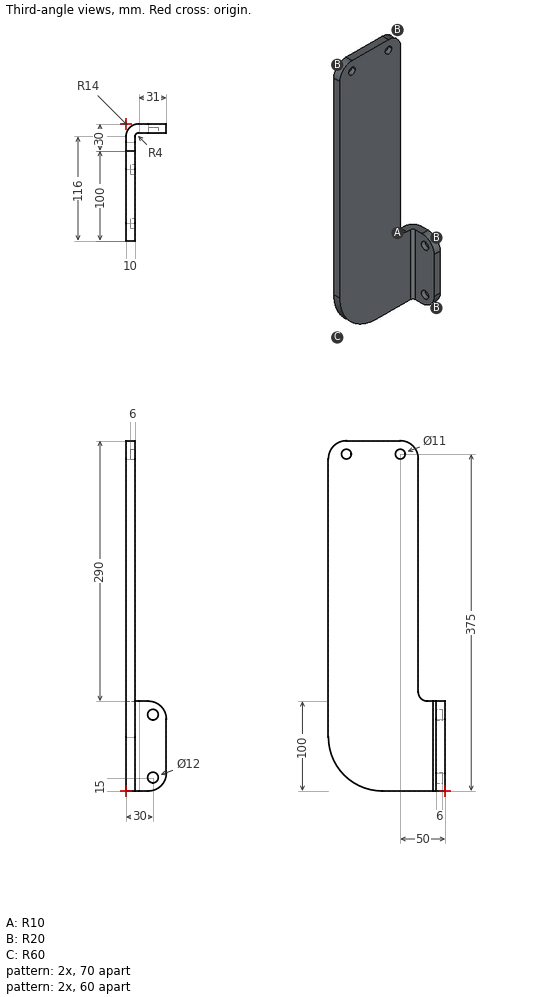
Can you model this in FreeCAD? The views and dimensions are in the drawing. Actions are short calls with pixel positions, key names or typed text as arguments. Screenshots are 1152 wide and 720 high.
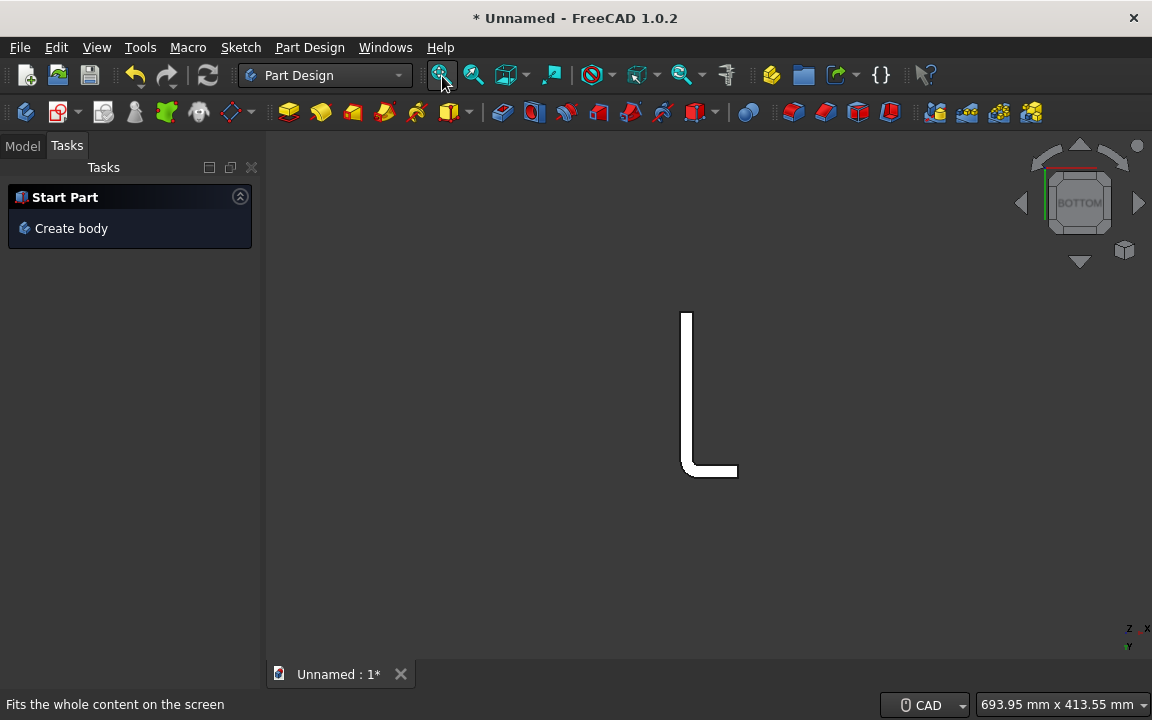
scroll(687, 439, up, 6)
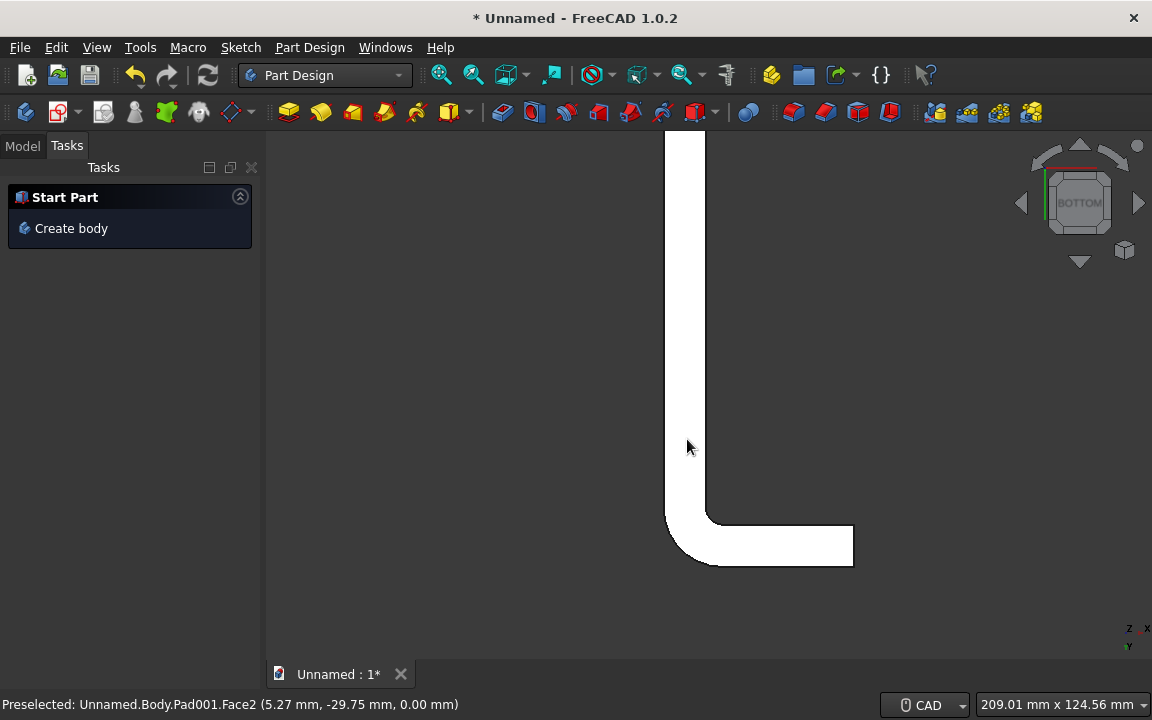
click(442, 76)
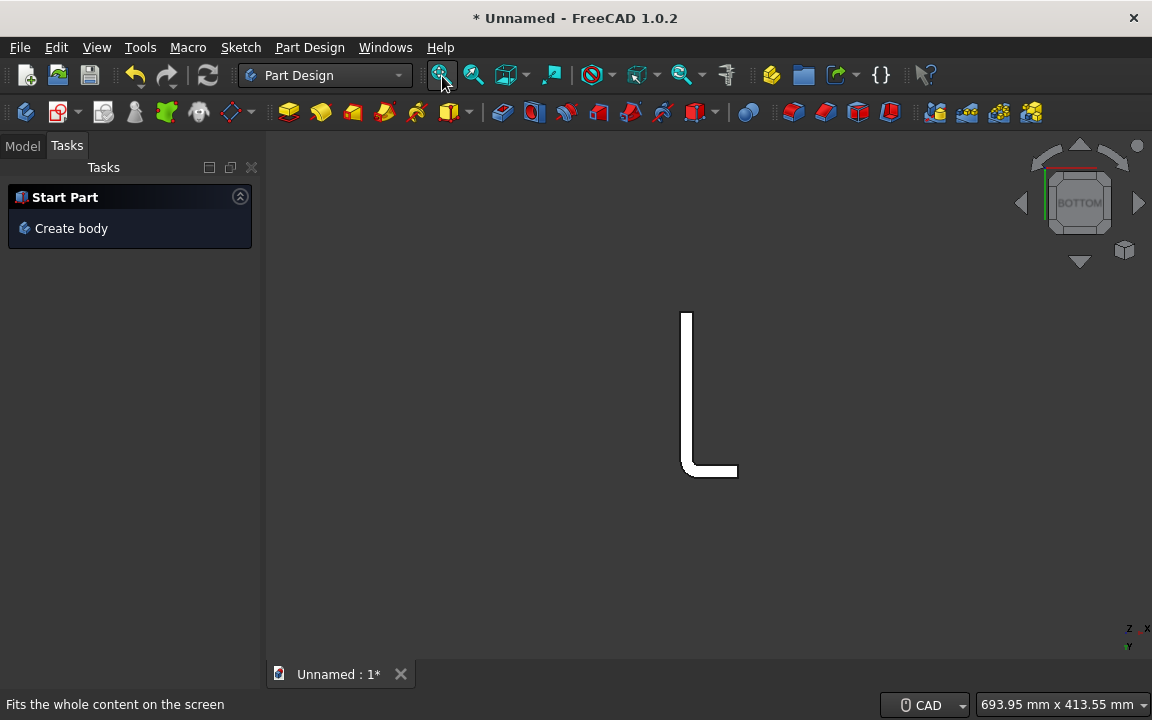
key(4)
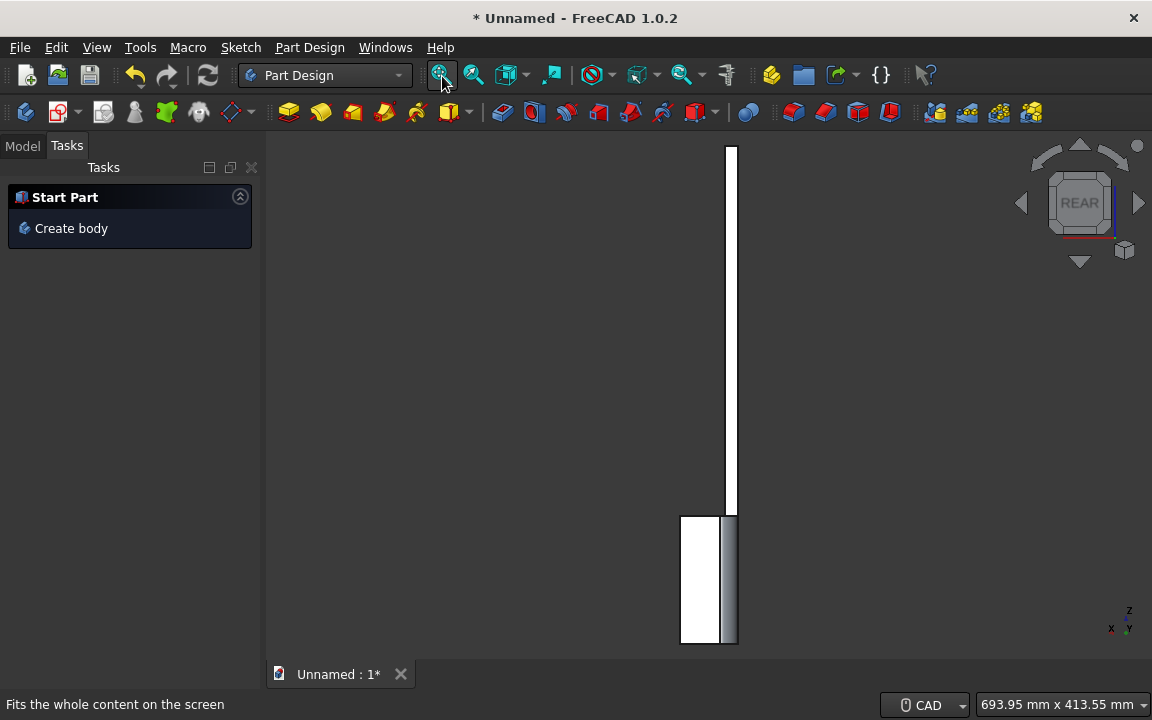
scroll(731, 515, up, 6)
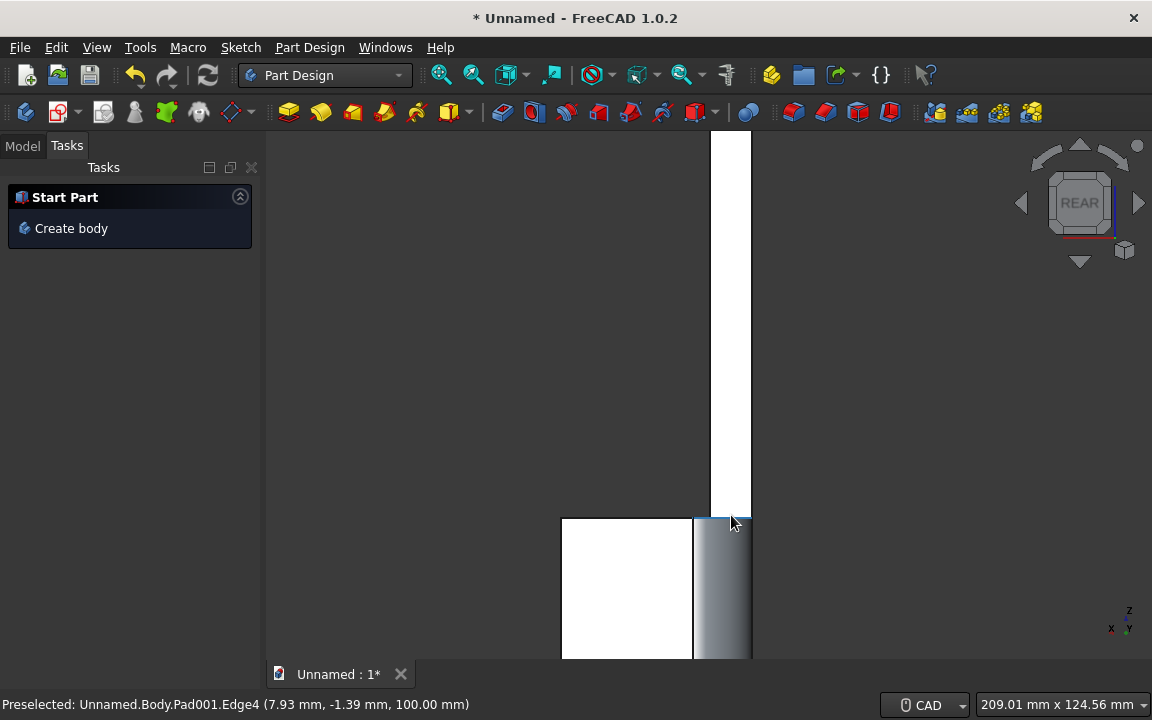
click(442, 76)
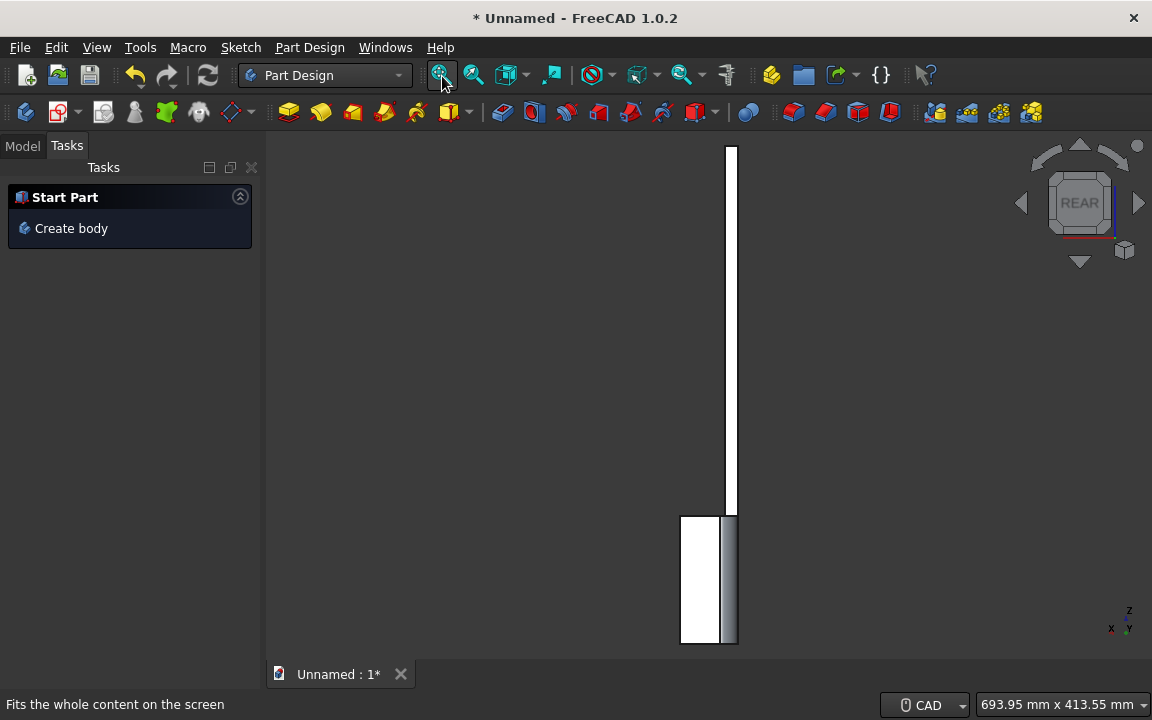
key(6)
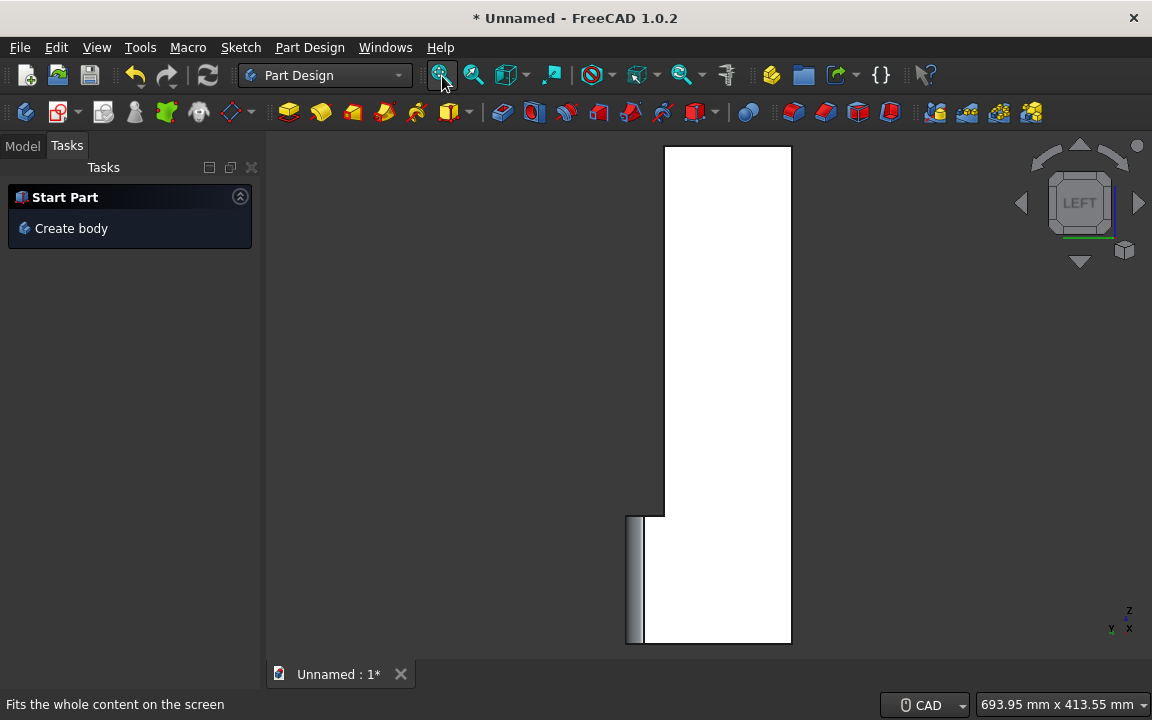
scroll(664, 515, up, 6)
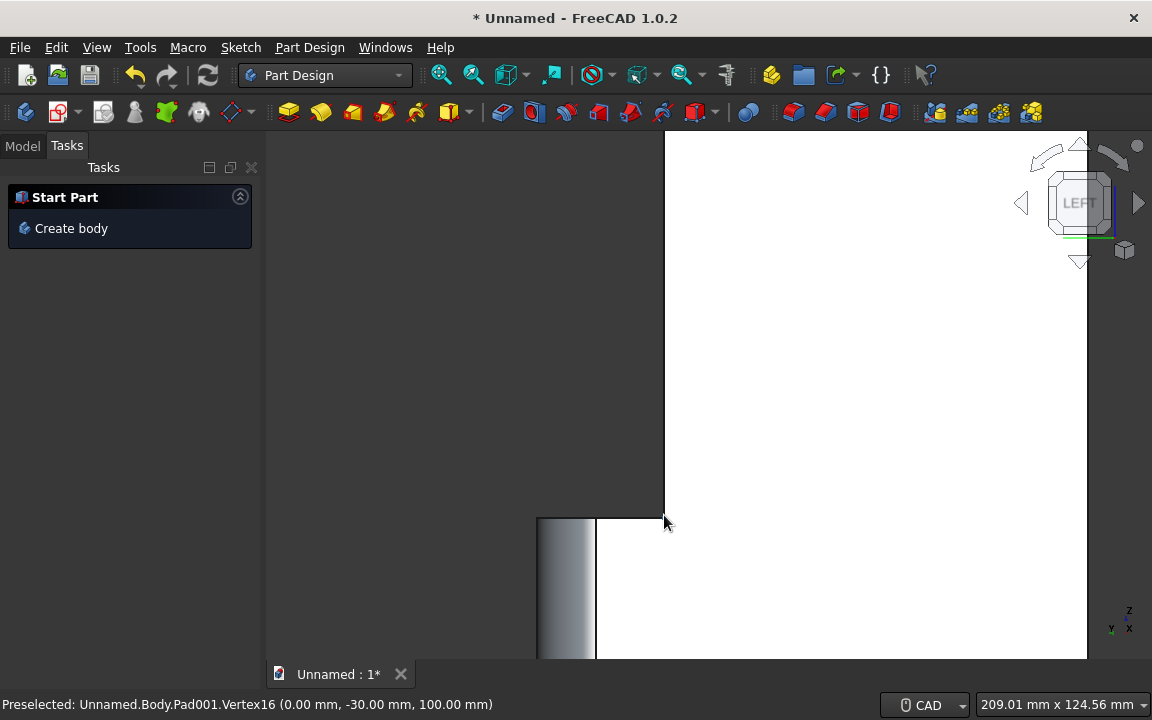
click(442, 76)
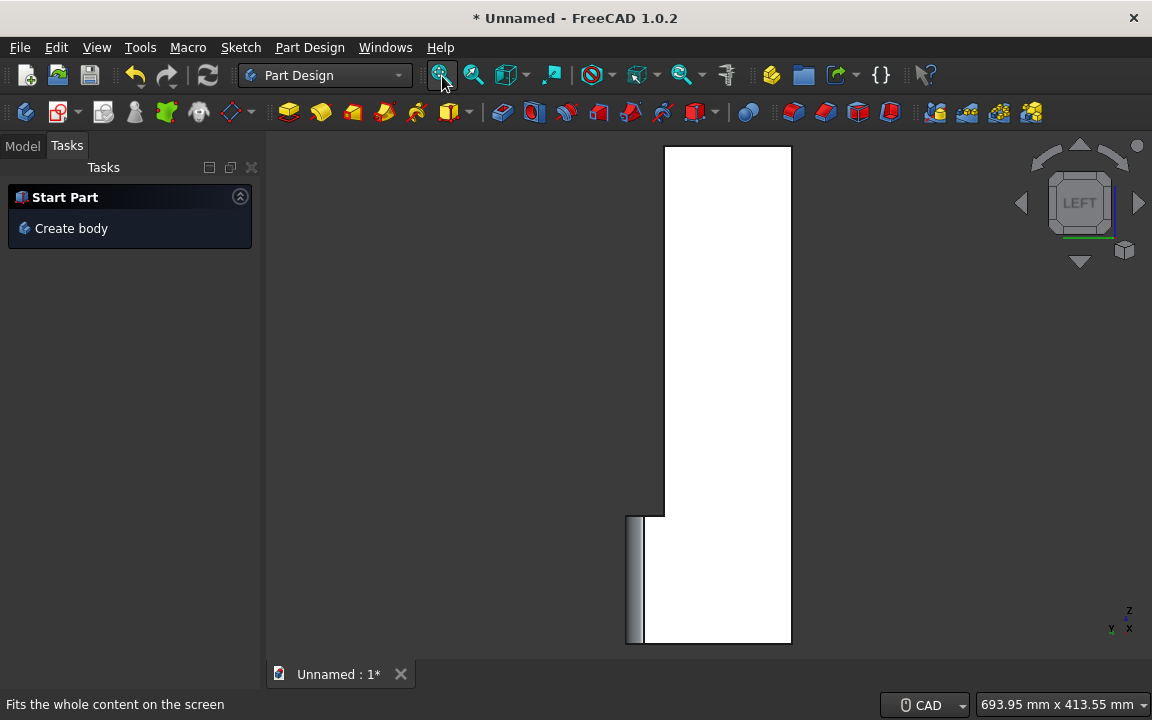
key(v)
key(3)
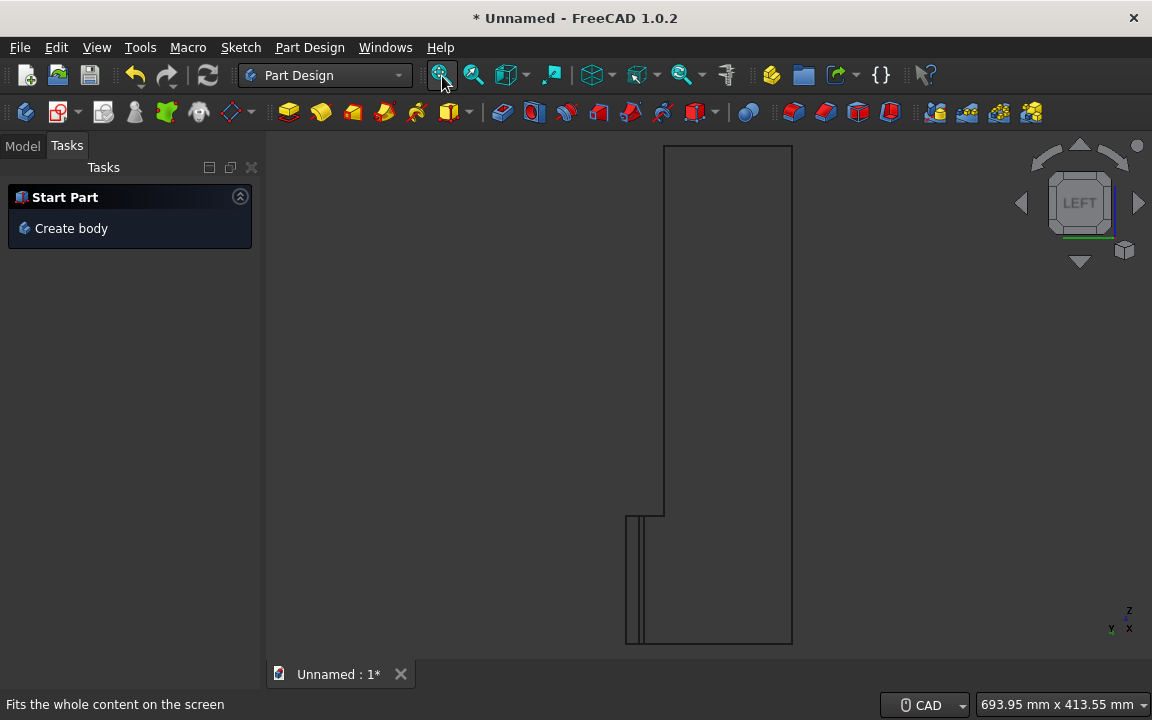
key(0)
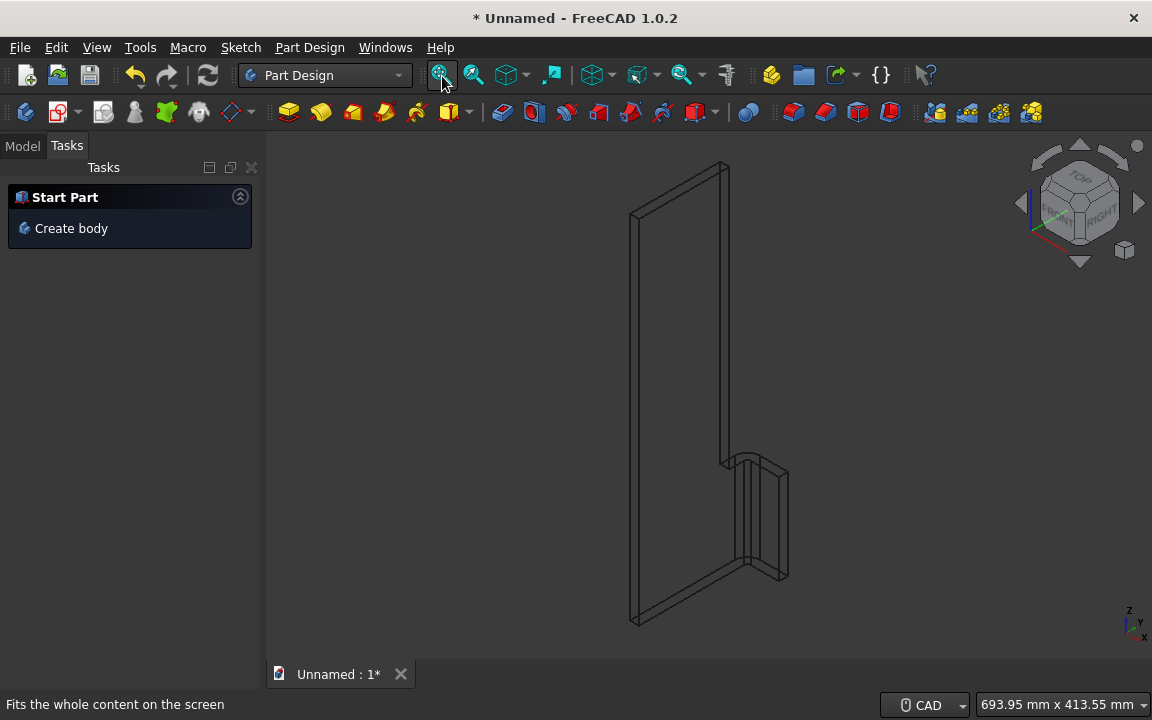
click(723, 465)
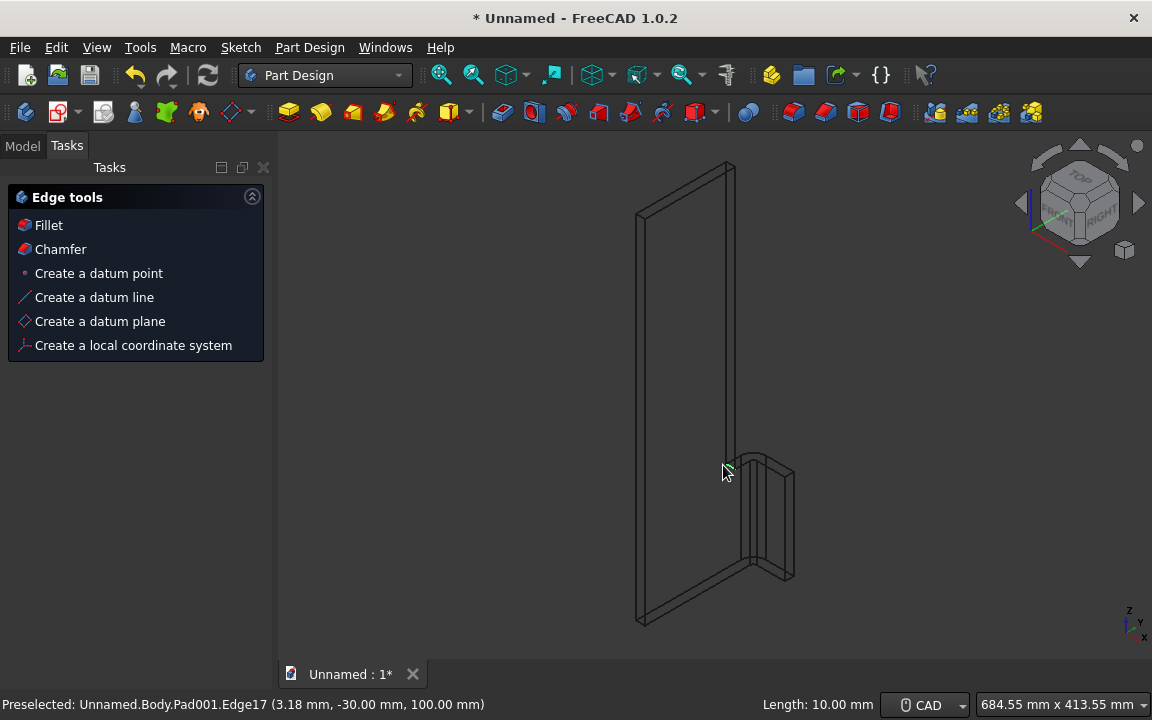
key(v)
key(1)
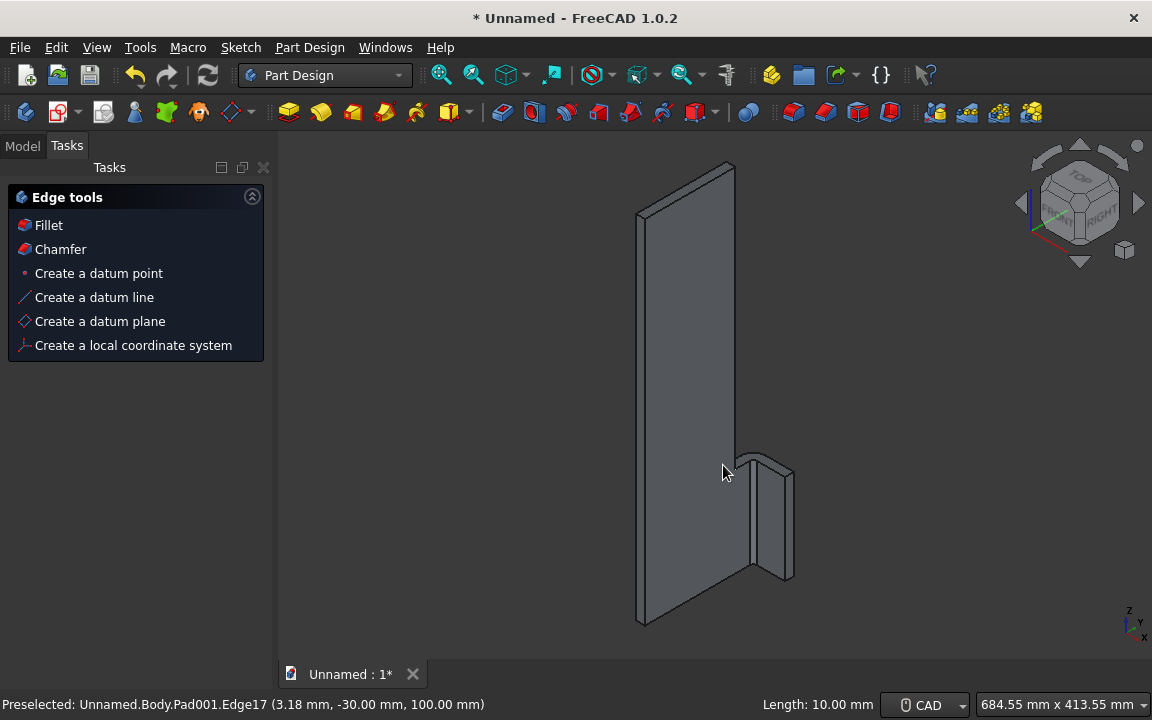
click(794, 112)